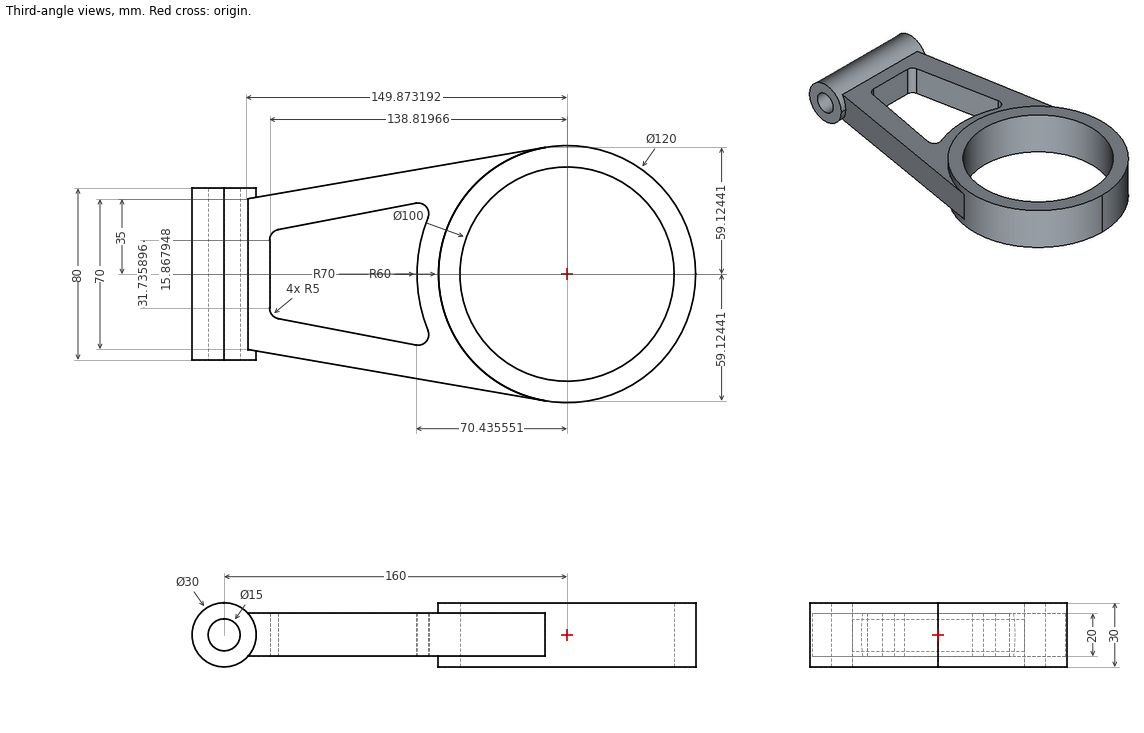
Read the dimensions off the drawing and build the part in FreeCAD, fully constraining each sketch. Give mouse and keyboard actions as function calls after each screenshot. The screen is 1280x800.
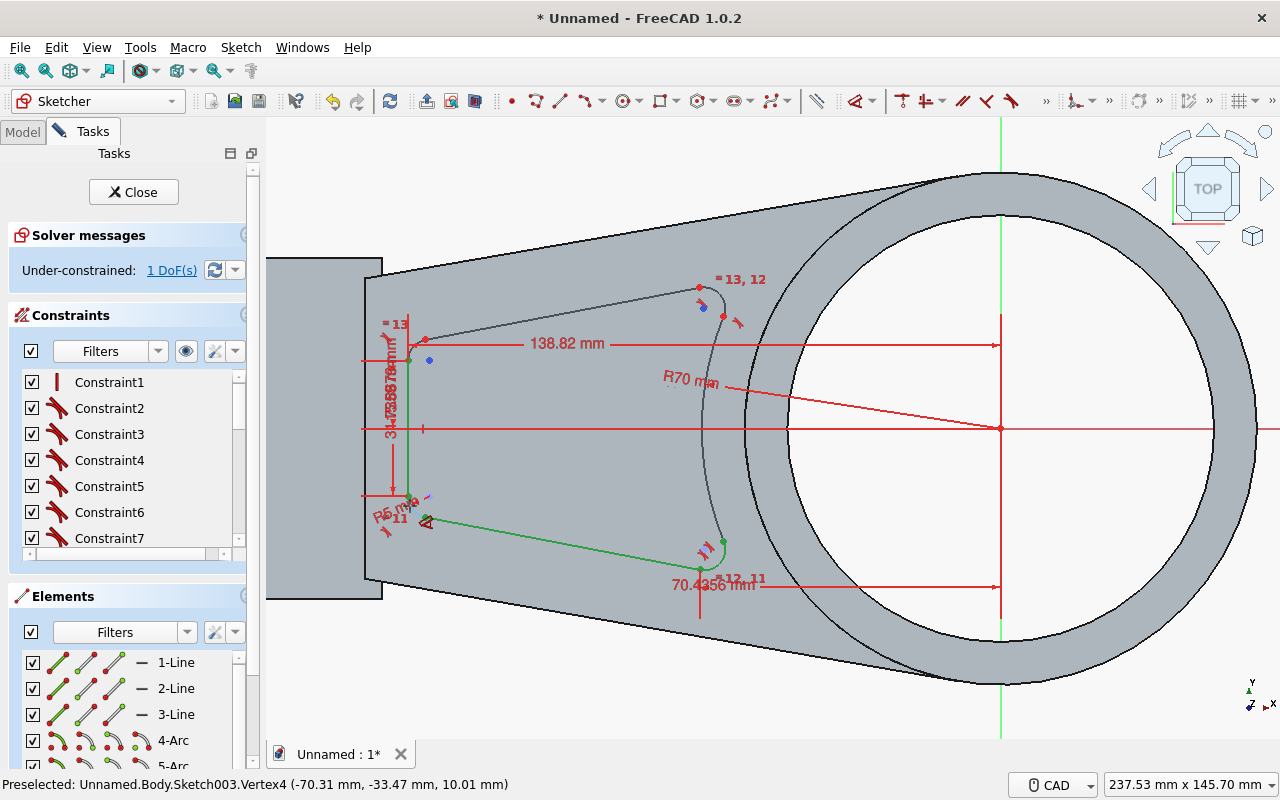
click(700, 288)
click(850, 254)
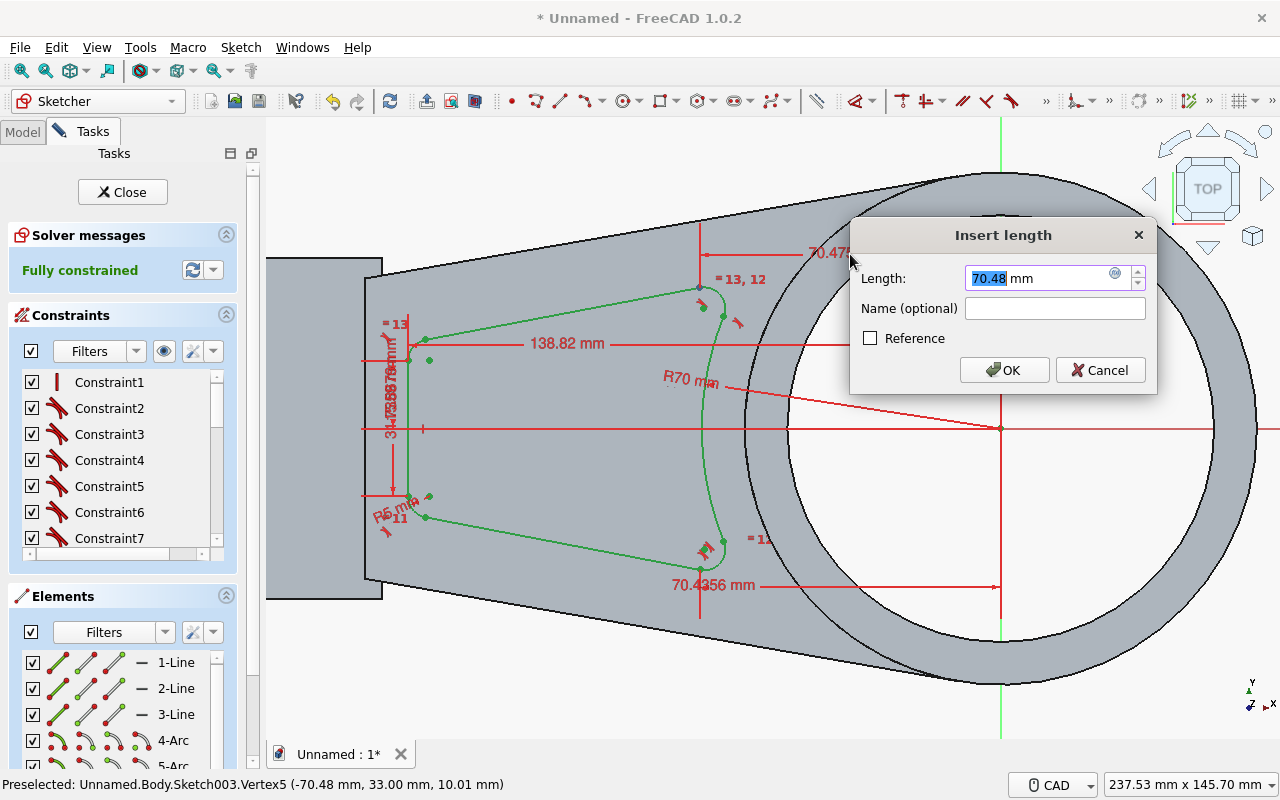
text(70.435551)
key(Return)
key(Escape)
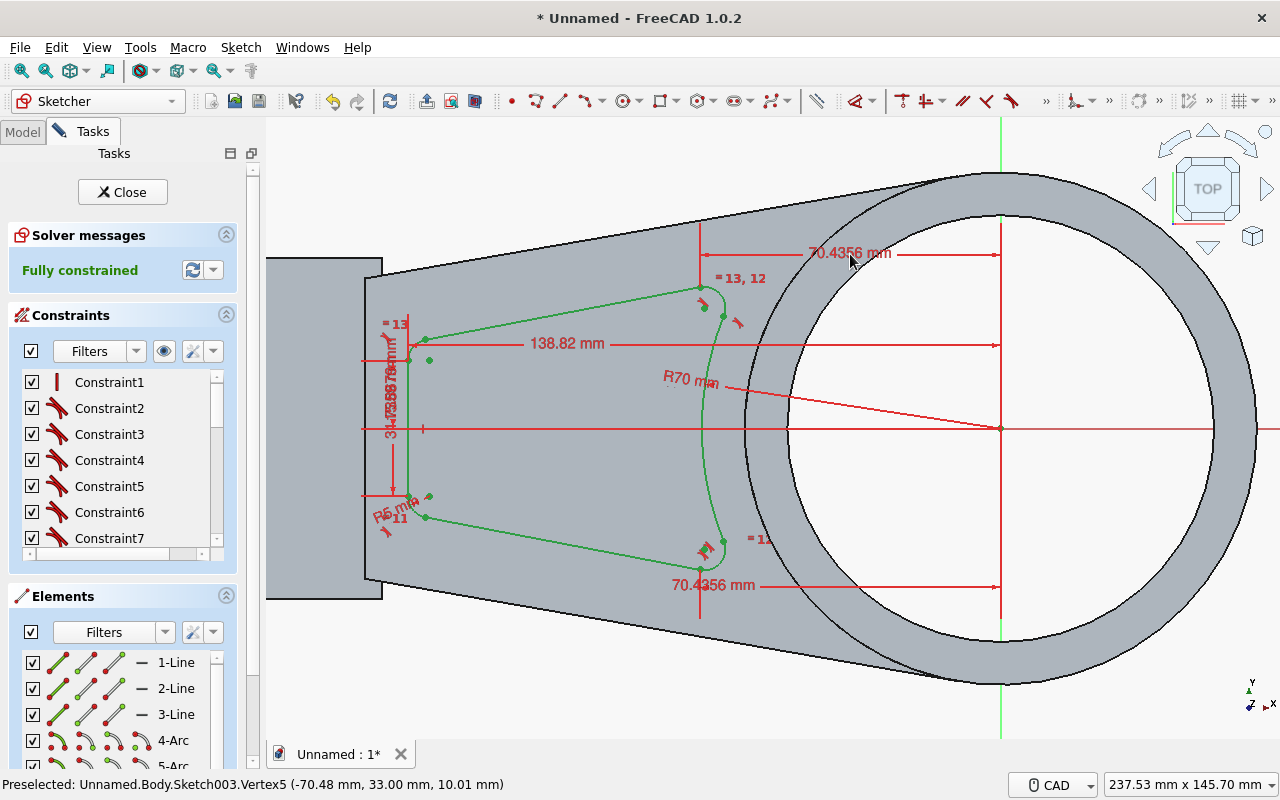
click(123, 192)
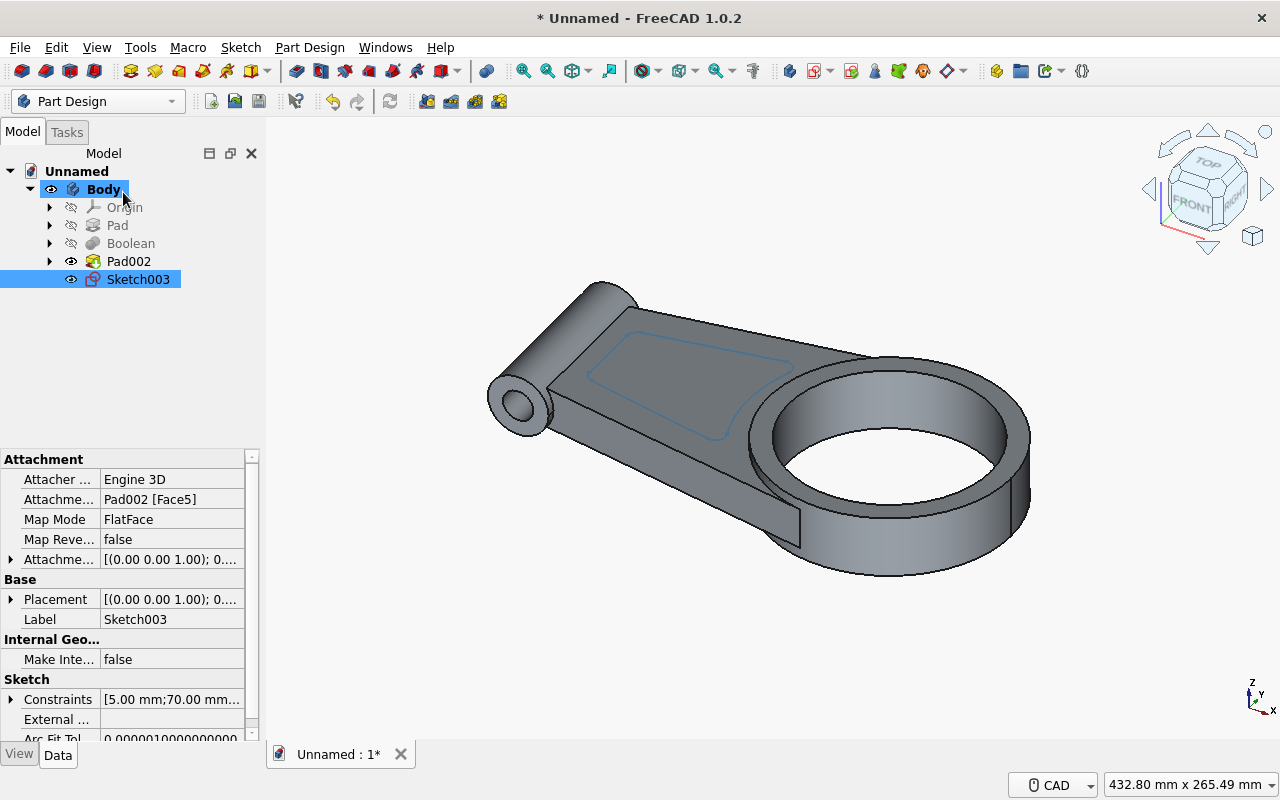
click(298, 72)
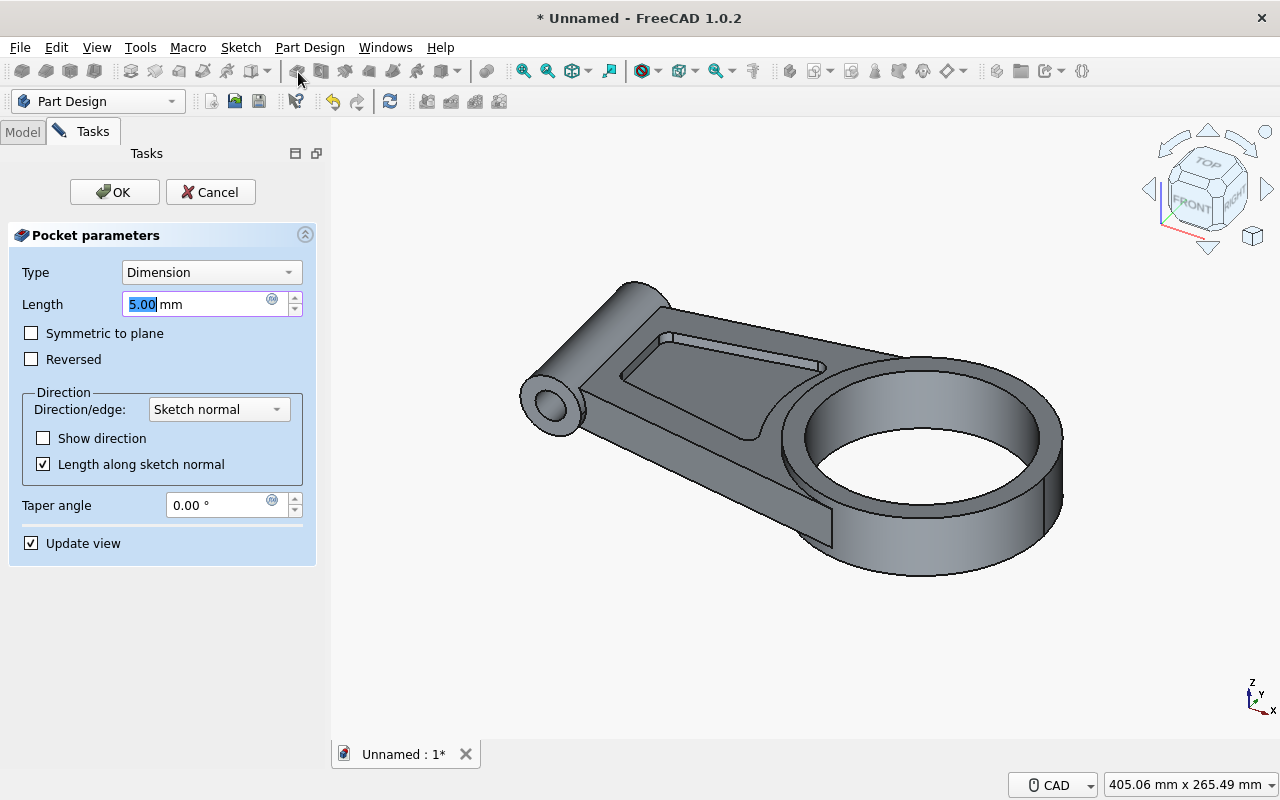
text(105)
key(Tab)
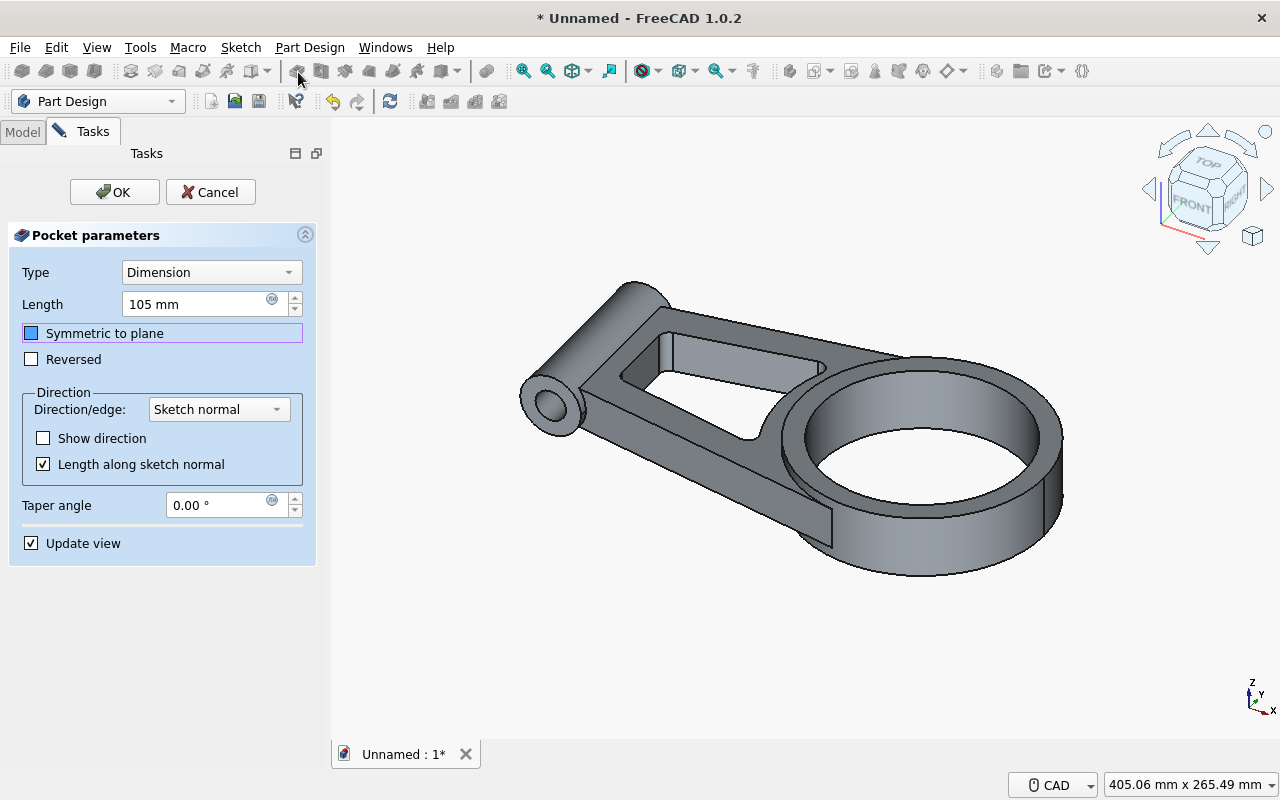
click(30, 333)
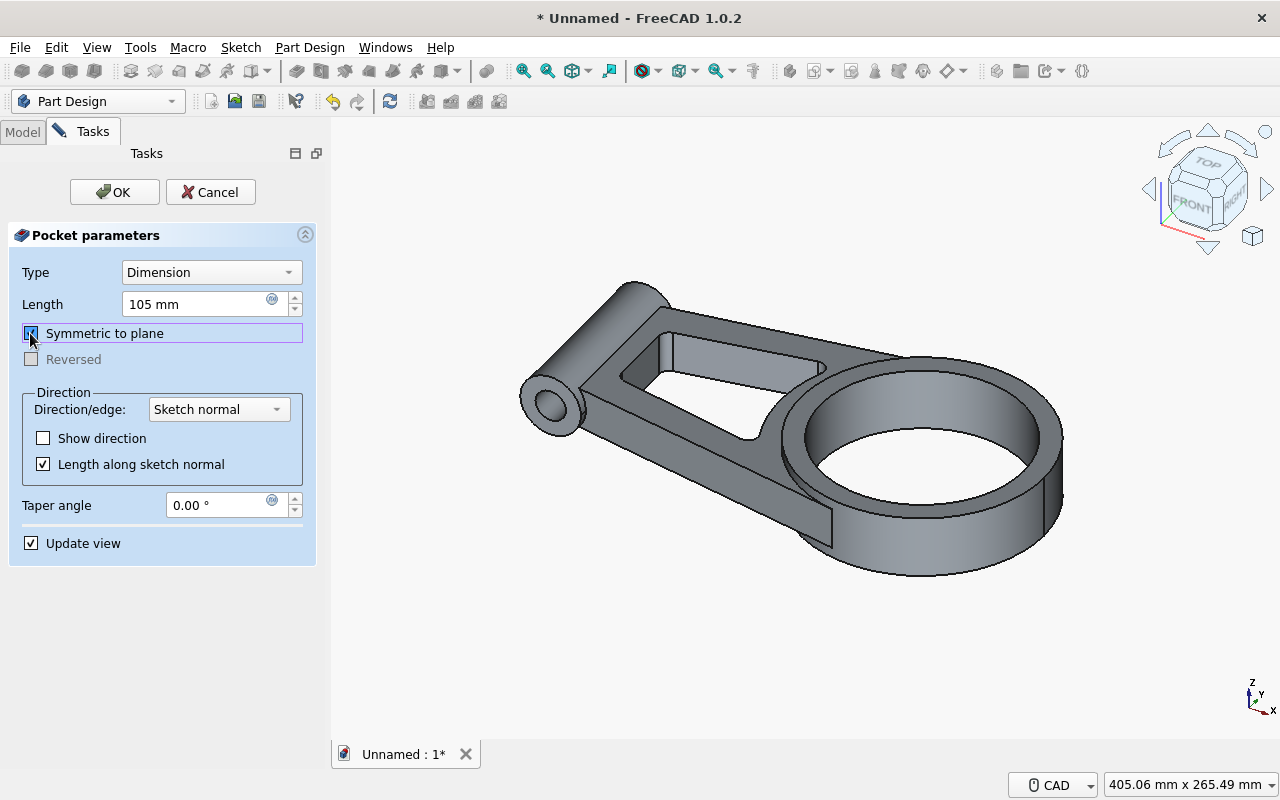
click(115, 192)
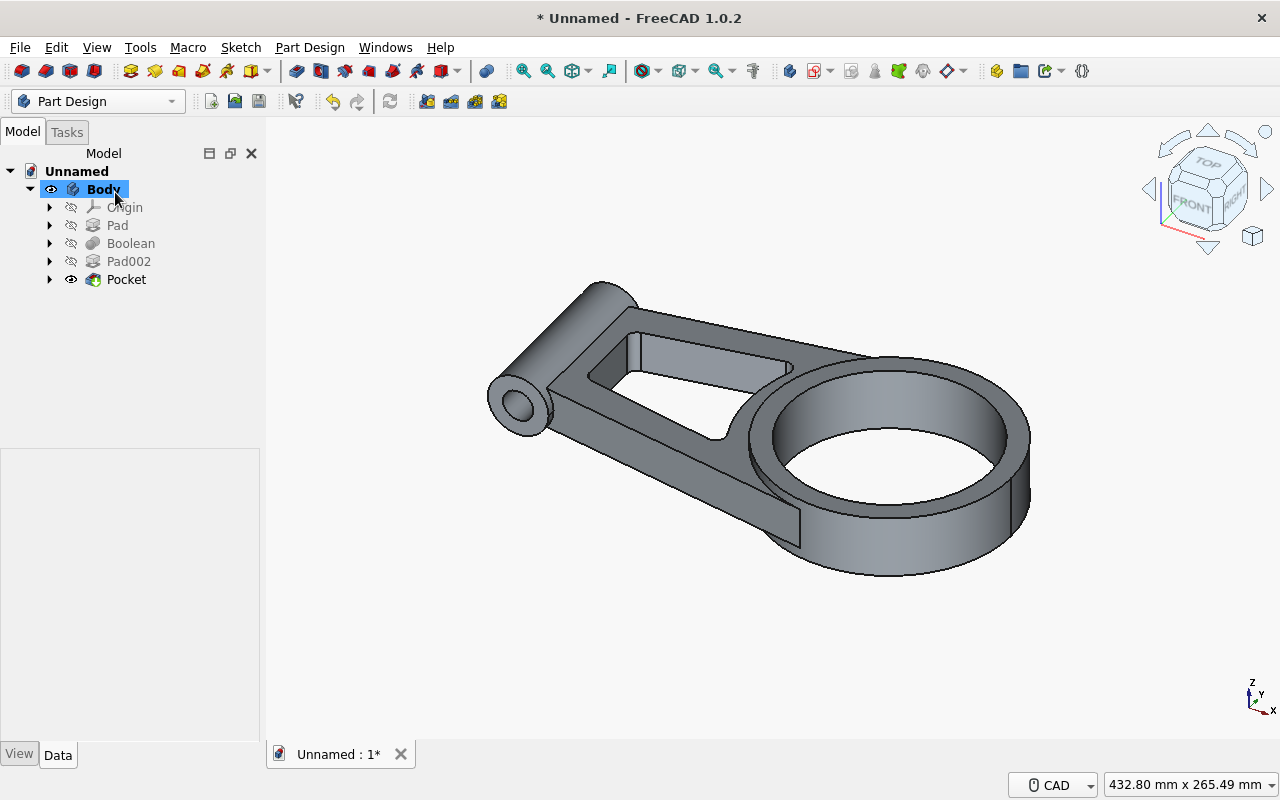
key(0)